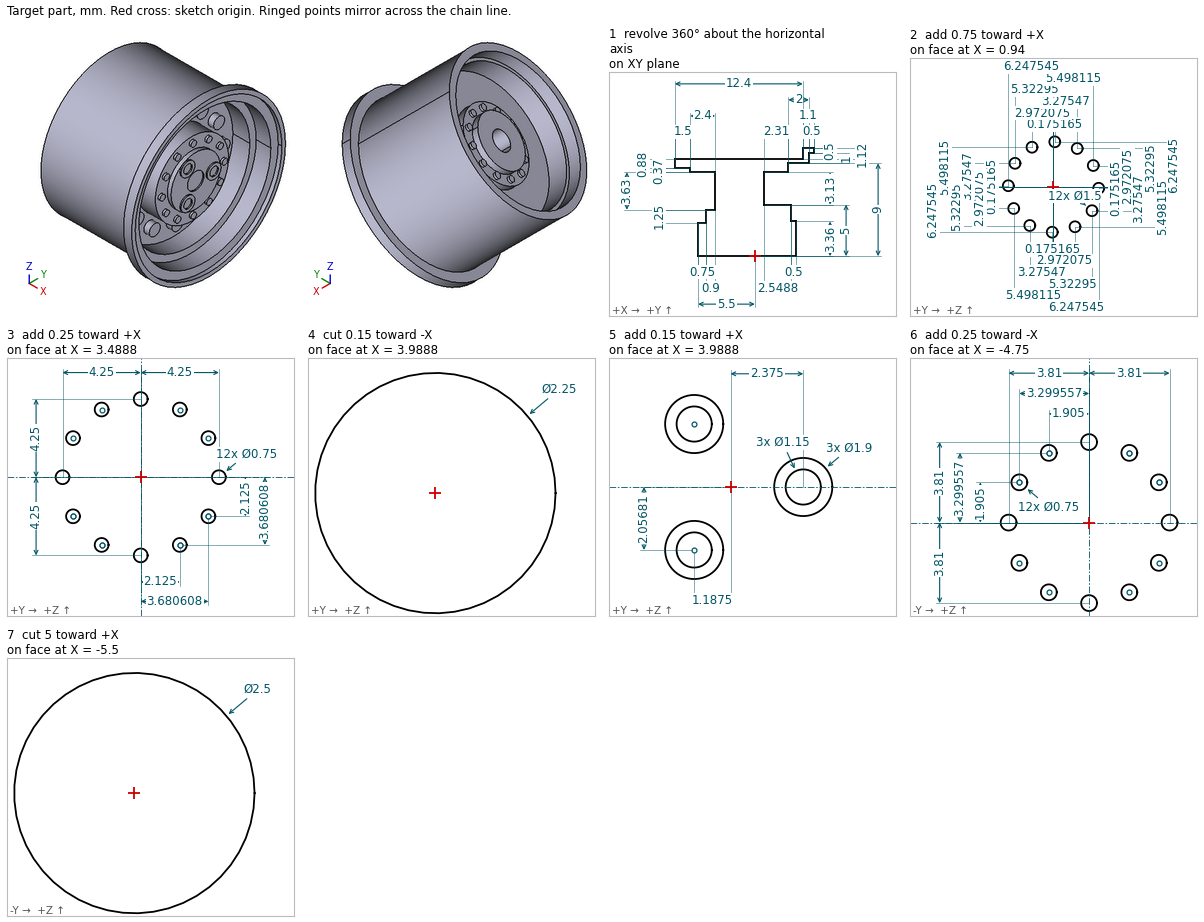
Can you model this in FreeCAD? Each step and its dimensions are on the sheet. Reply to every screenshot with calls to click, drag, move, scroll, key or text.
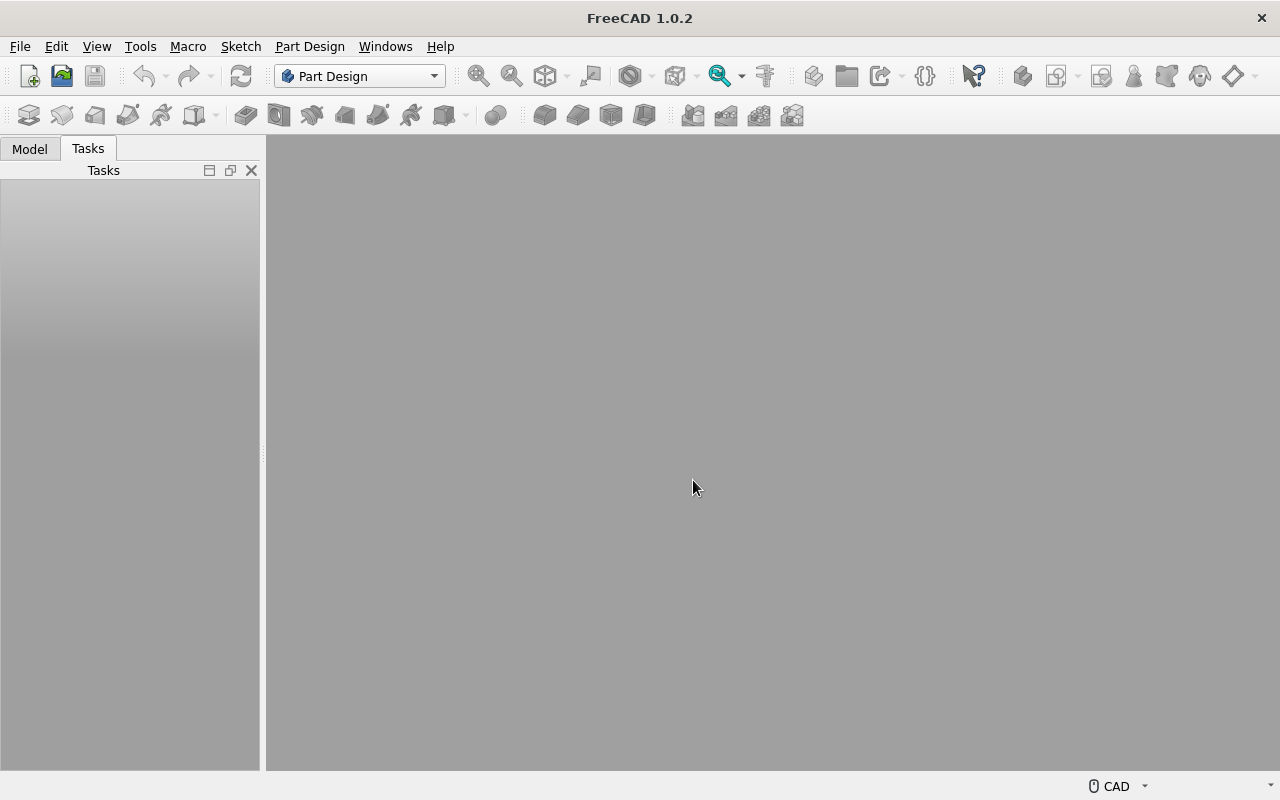
click(29, 76)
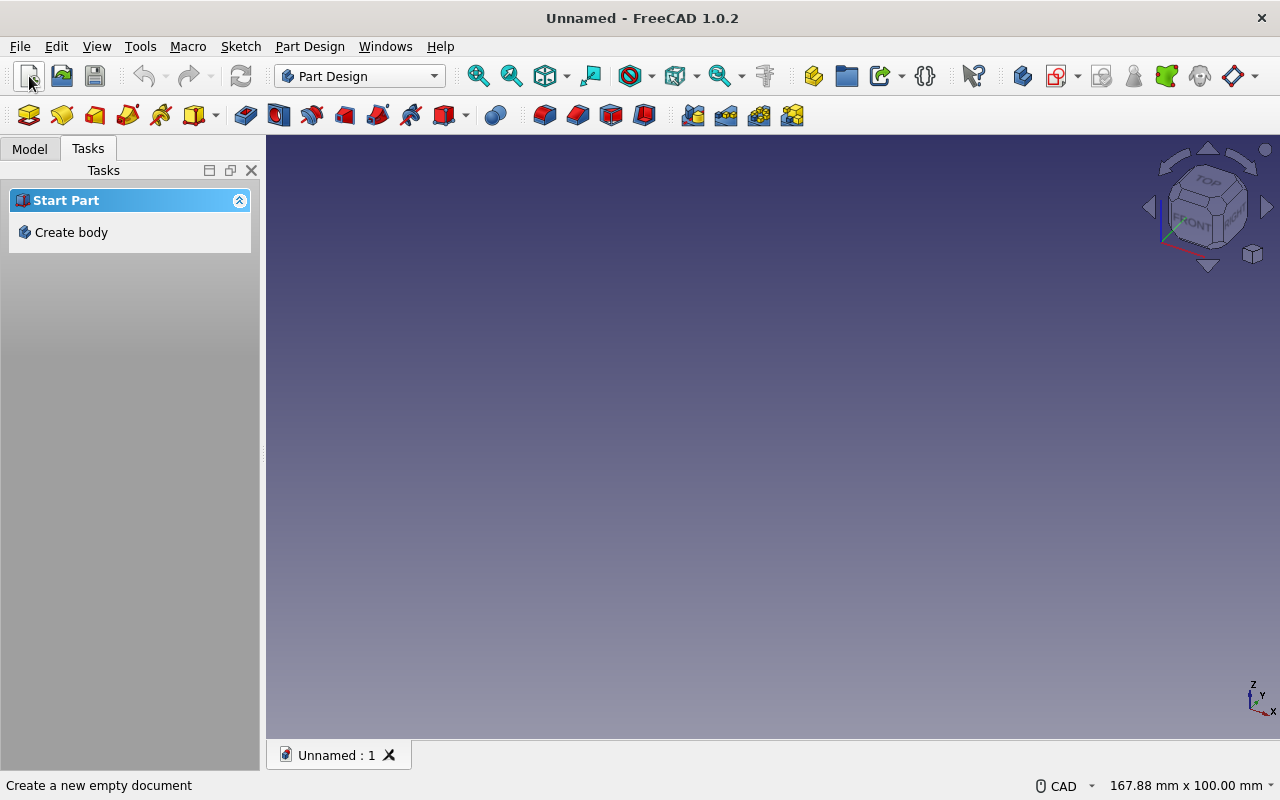
click(1056, 76)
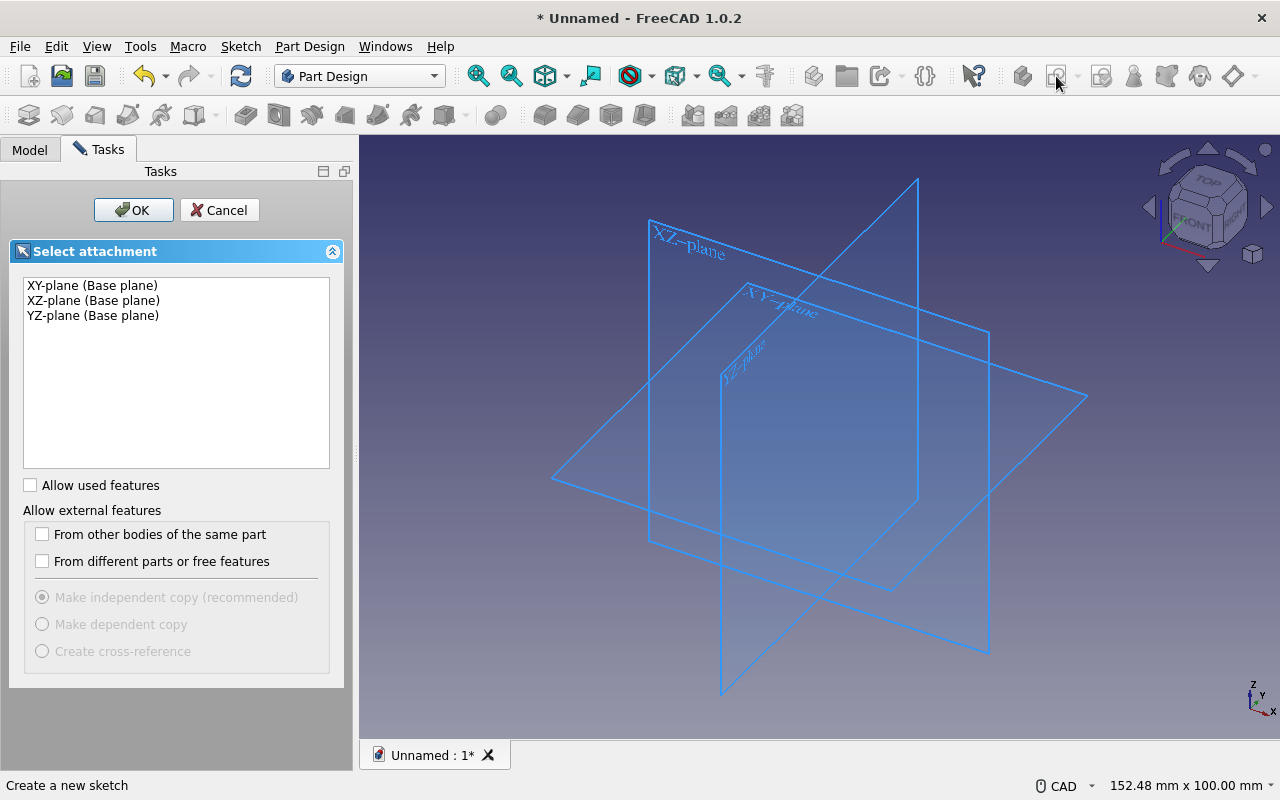
click(84, 286)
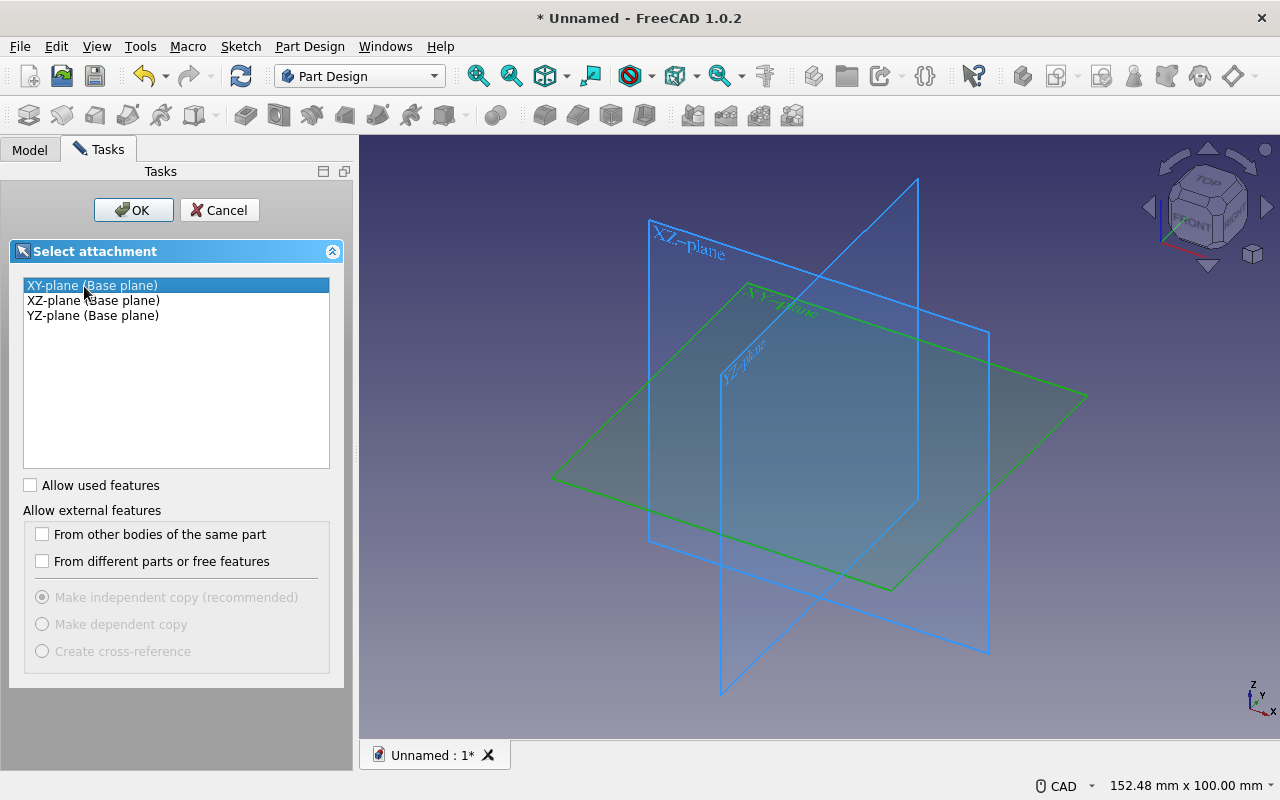
click(134, 210)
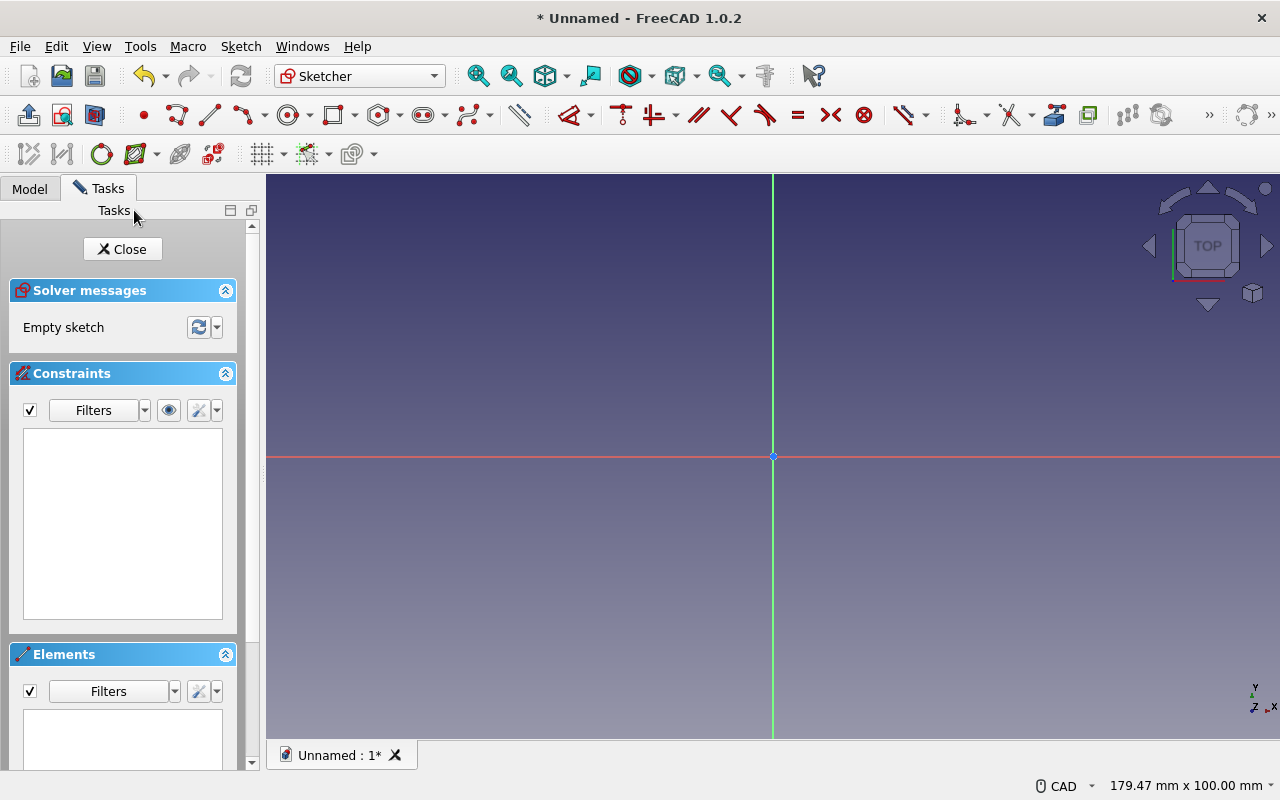
scroll(780, 421, up, 9)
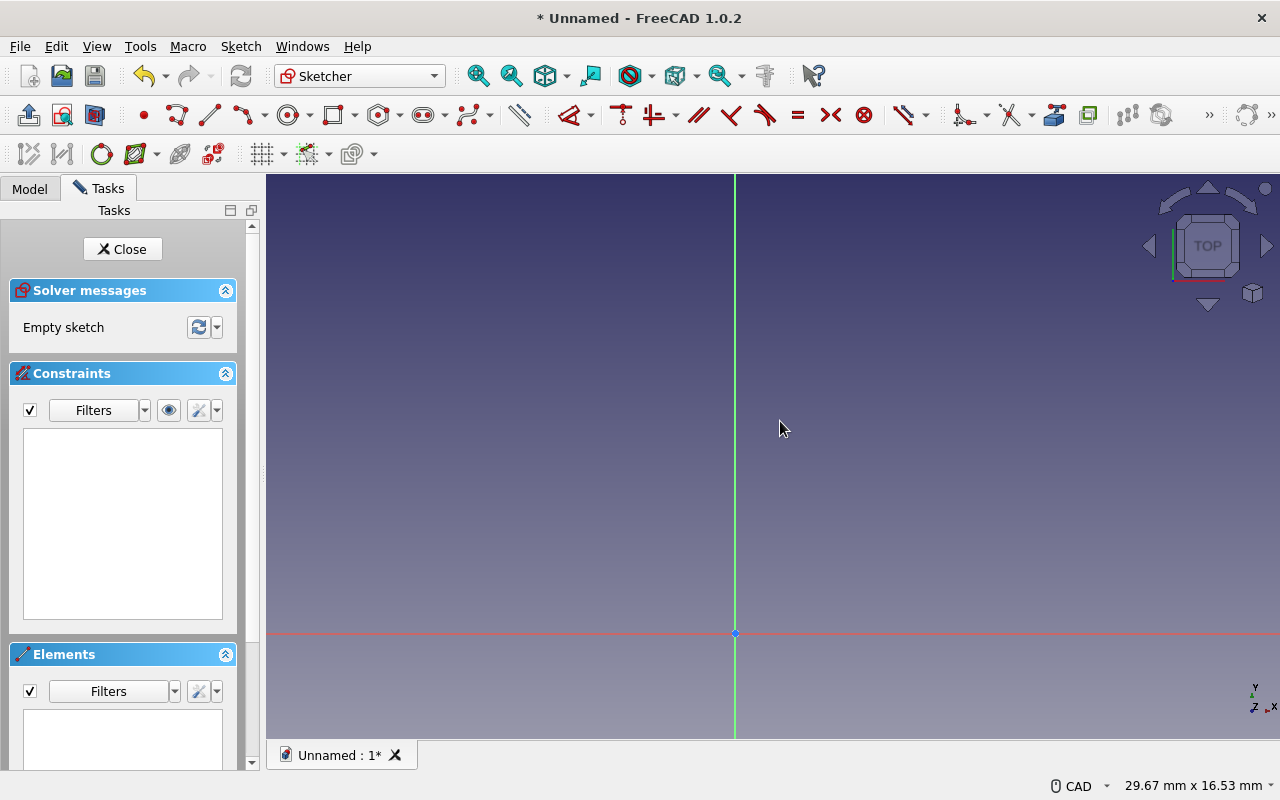
click(177, 116)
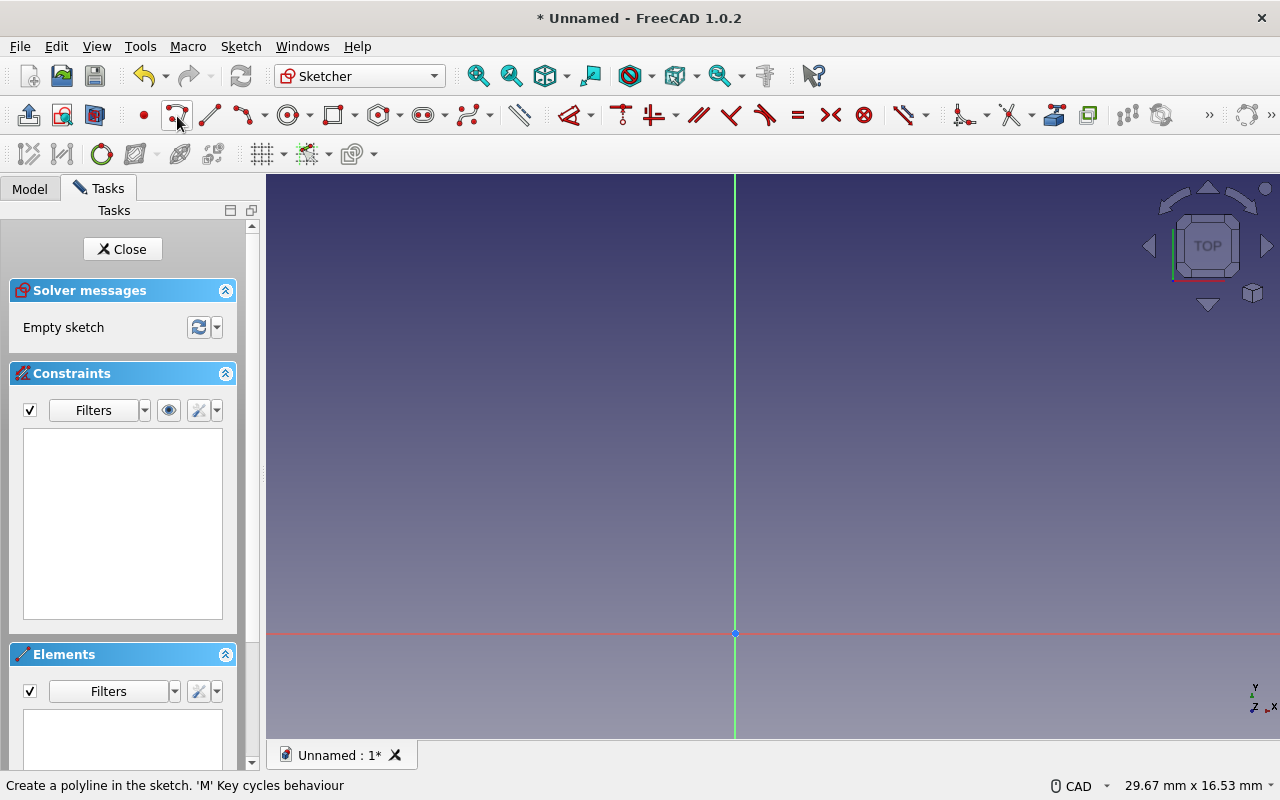
click(871, 634)
click(871, 519)
click(854, 519)
click(854, 463)
click(767, 463)
click(767, 356)
click(846, 356)
click(846, 326)
click(915, 326)
click(915, 292)
click(932, 292)
click(932, 275)
click(894, 275)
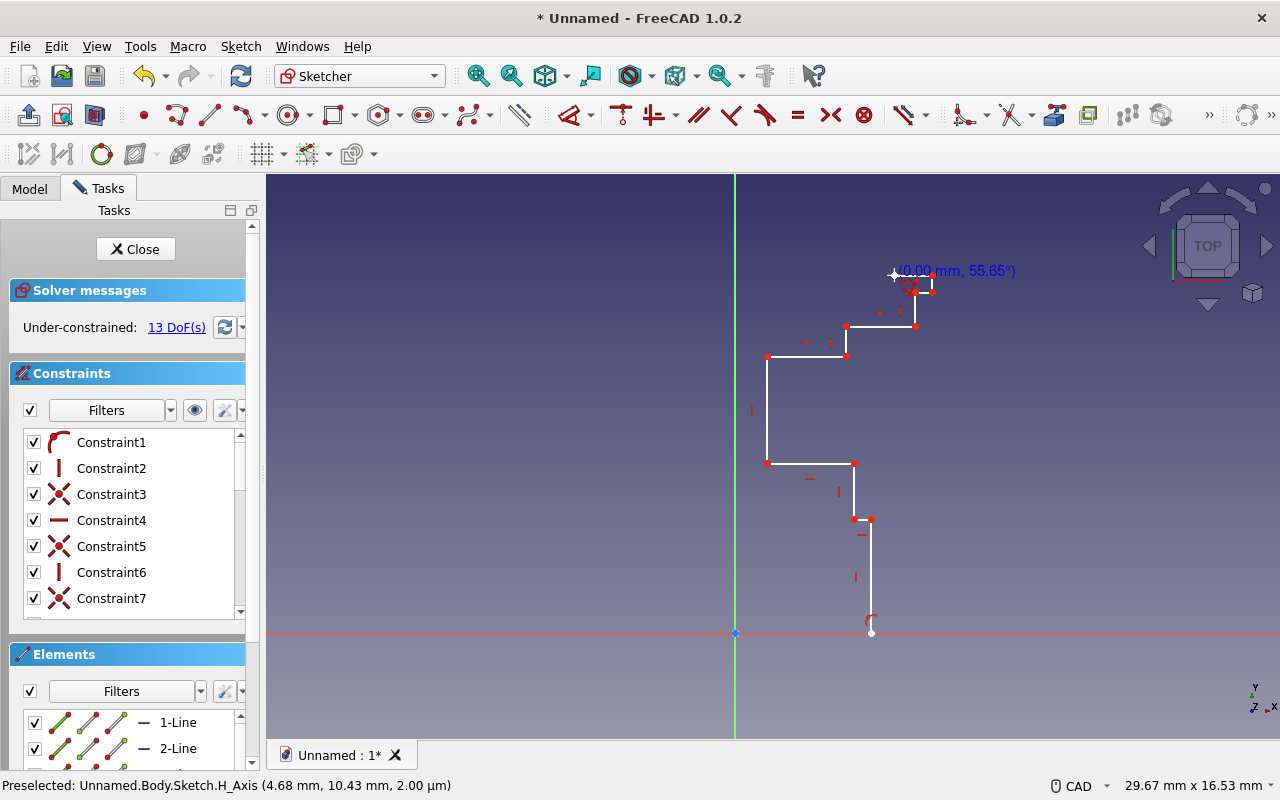
scroll(894, 313, up, 2)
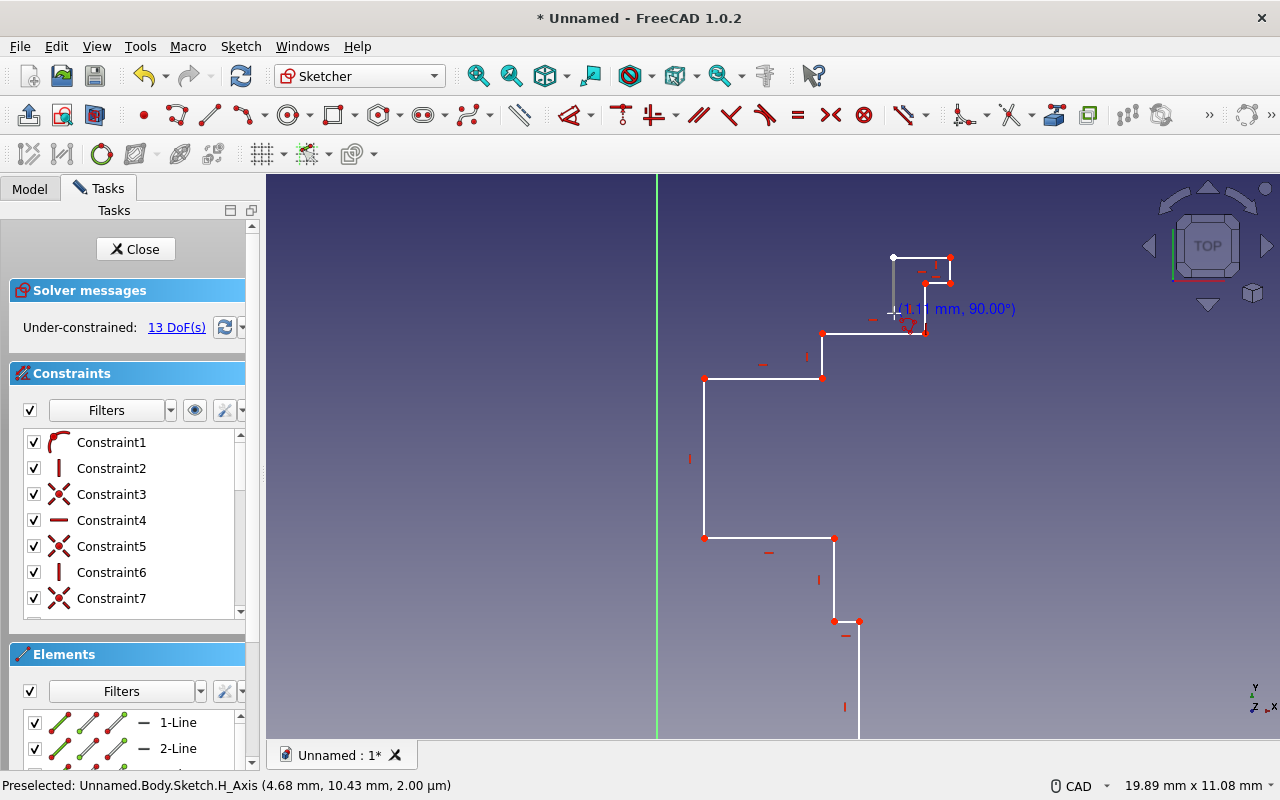
click(894, 313)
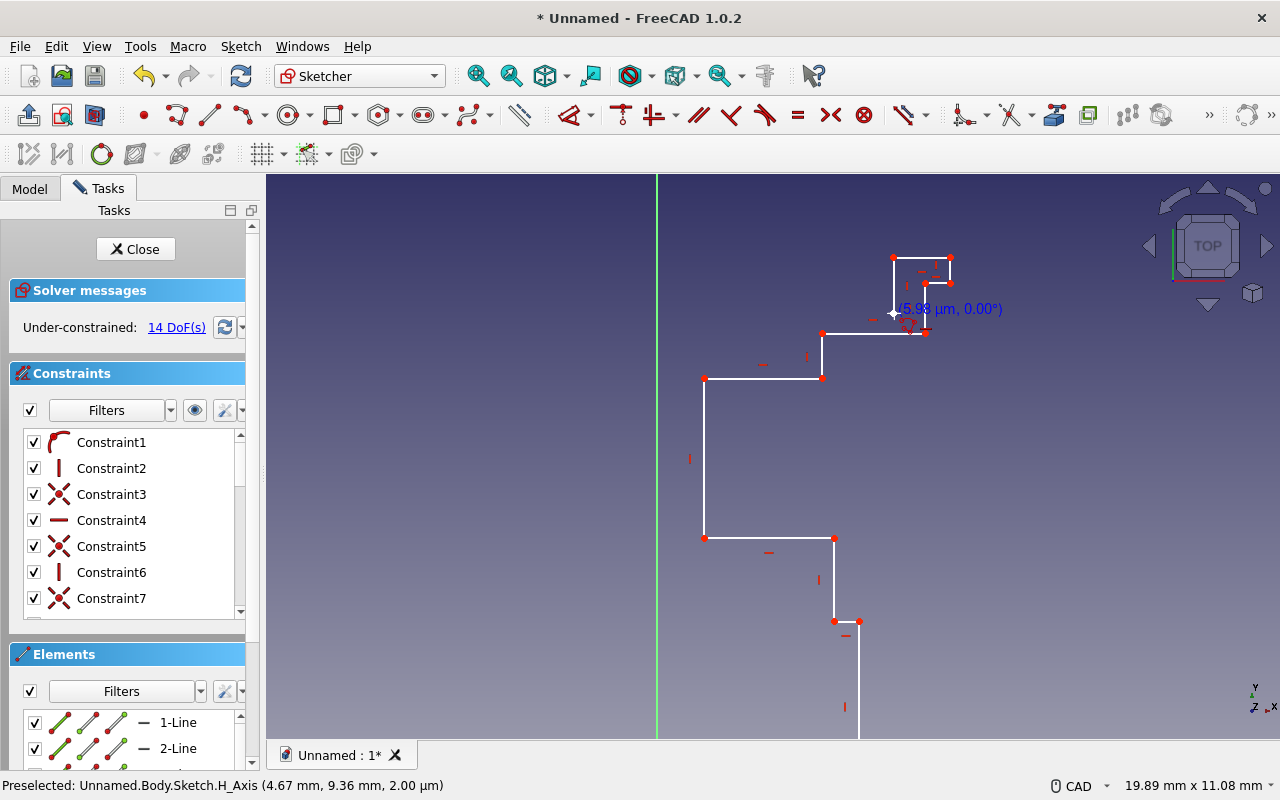
scroll(906, 321, down, 2)